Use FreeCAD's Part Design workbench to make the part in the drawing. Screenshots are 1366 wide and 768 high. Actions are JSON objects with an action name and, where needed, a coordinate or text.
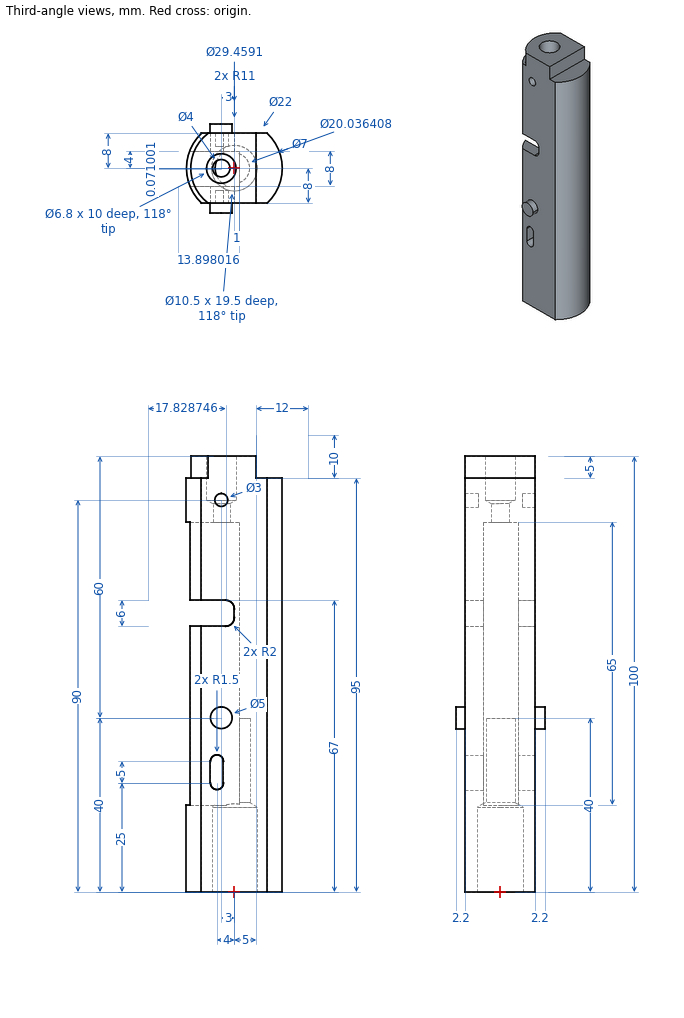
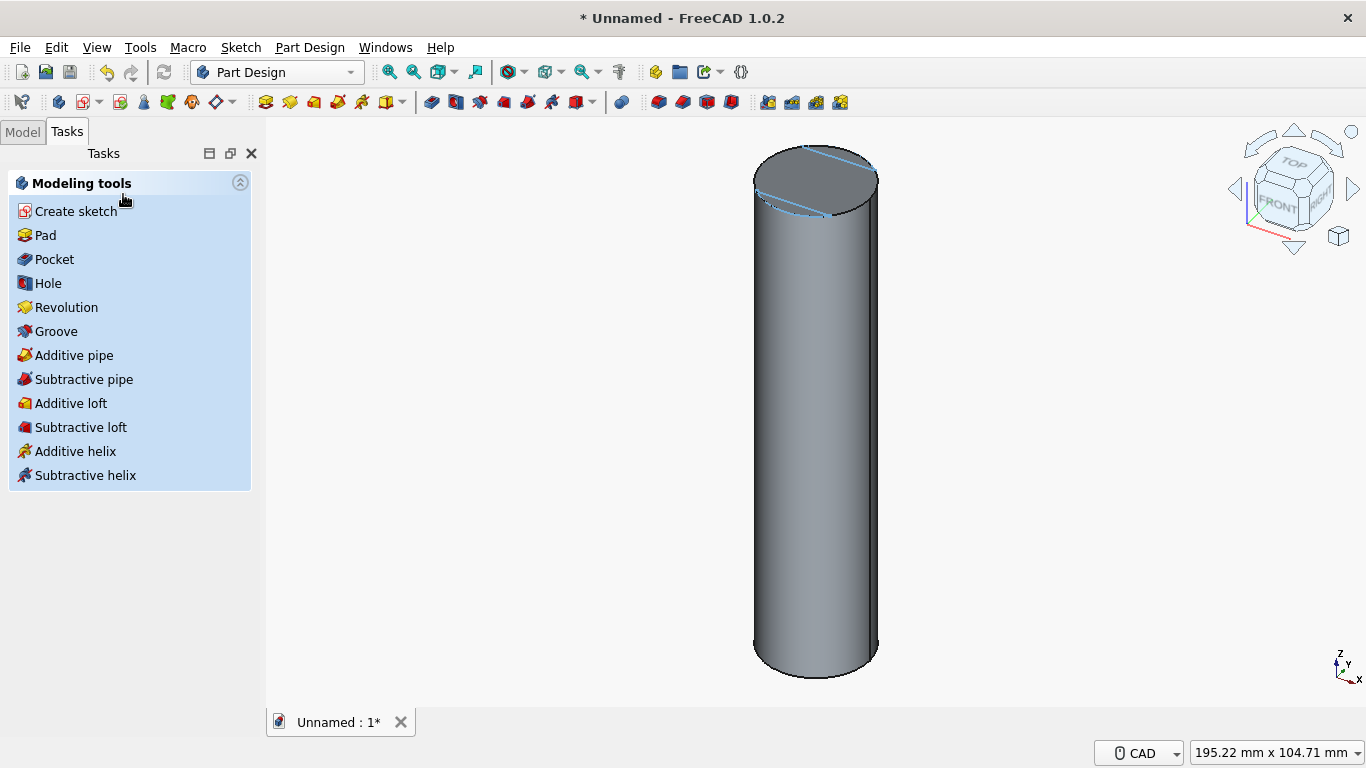
{"action": "left_click", "coordinate": [432, 102]}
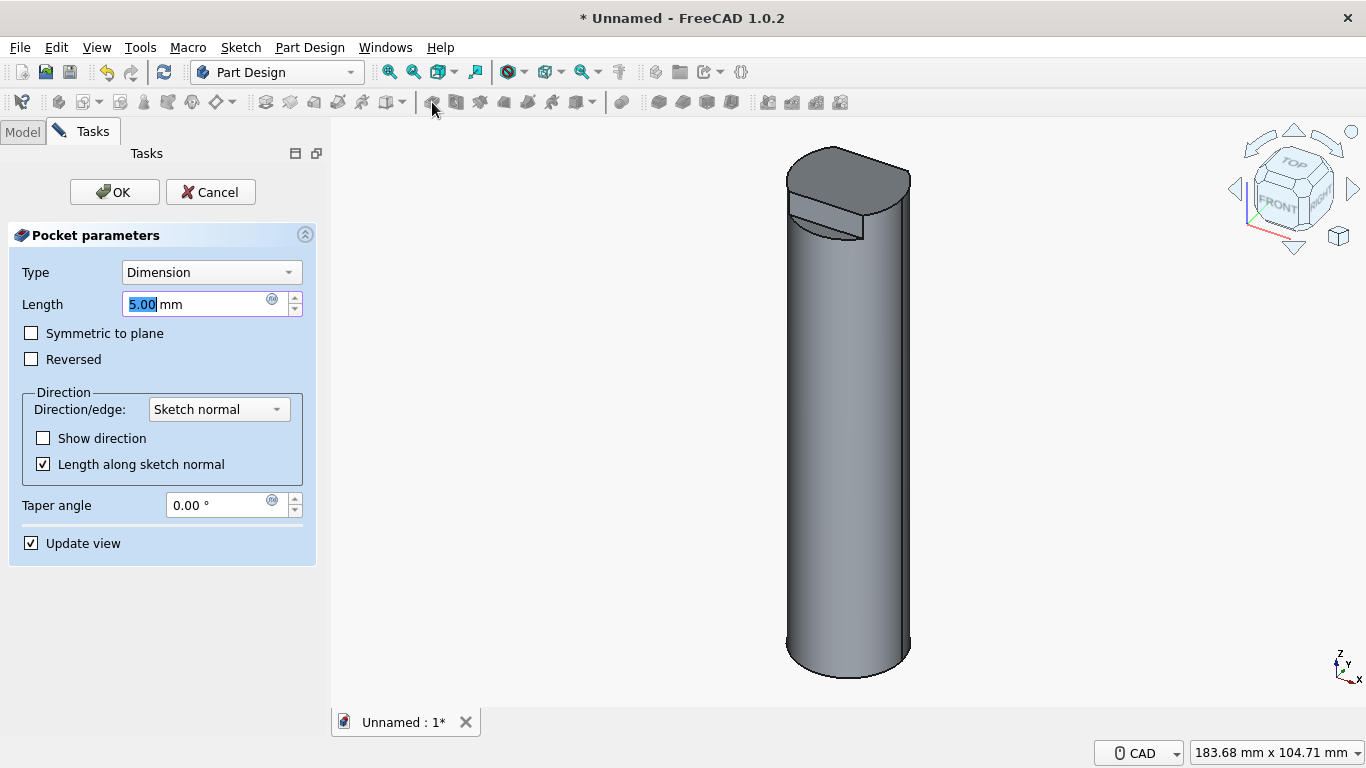
{"action": "left_click", "coordinate": [212, 272]}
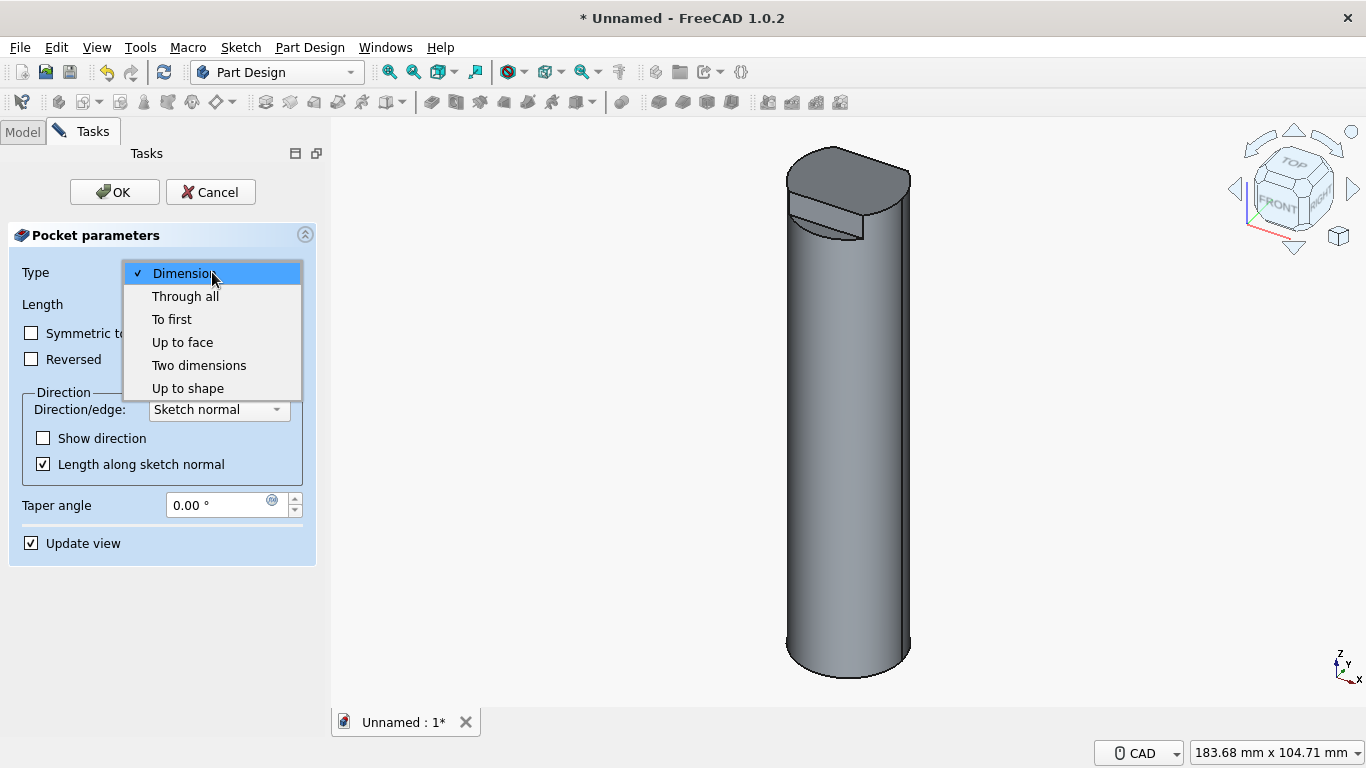
{"action": "left_click", "coordinate": [212, 296]}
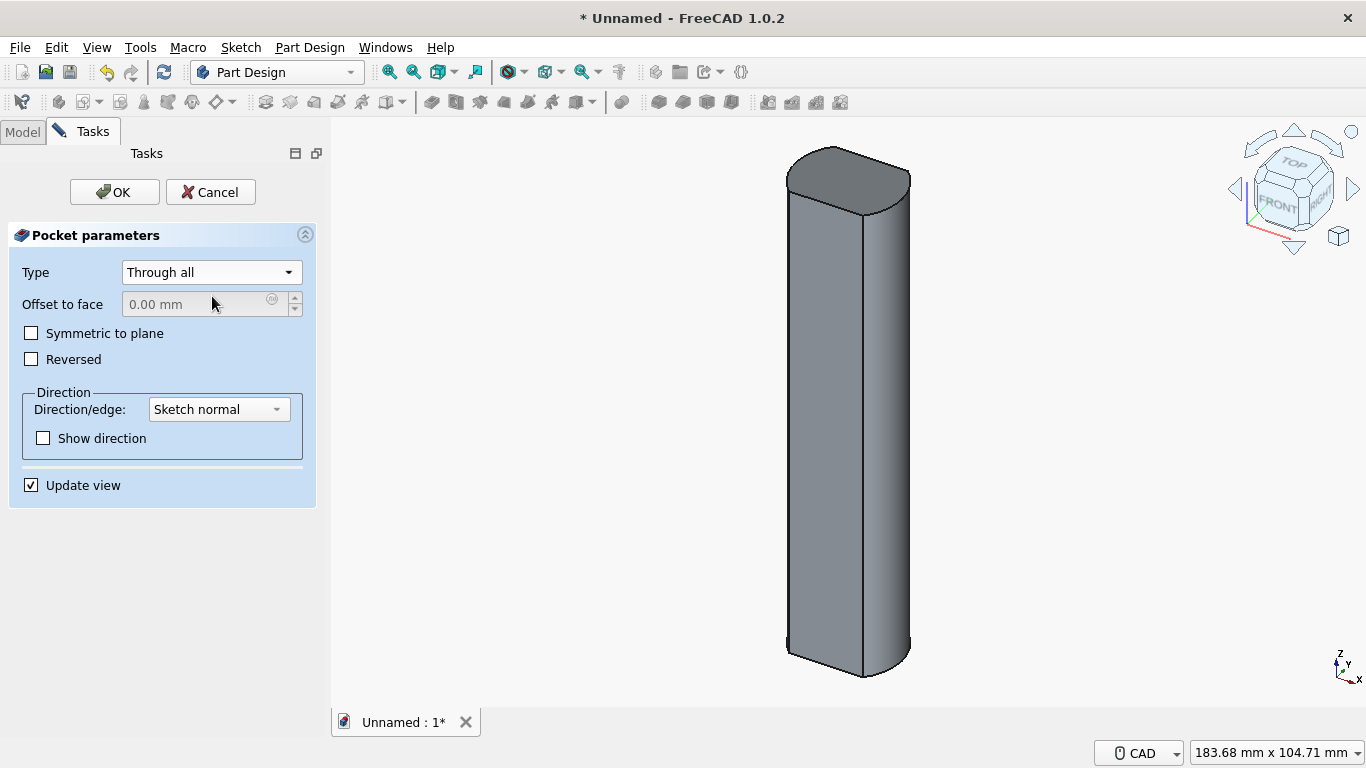
{"action": "left_click", "coordinate": [115, 192]}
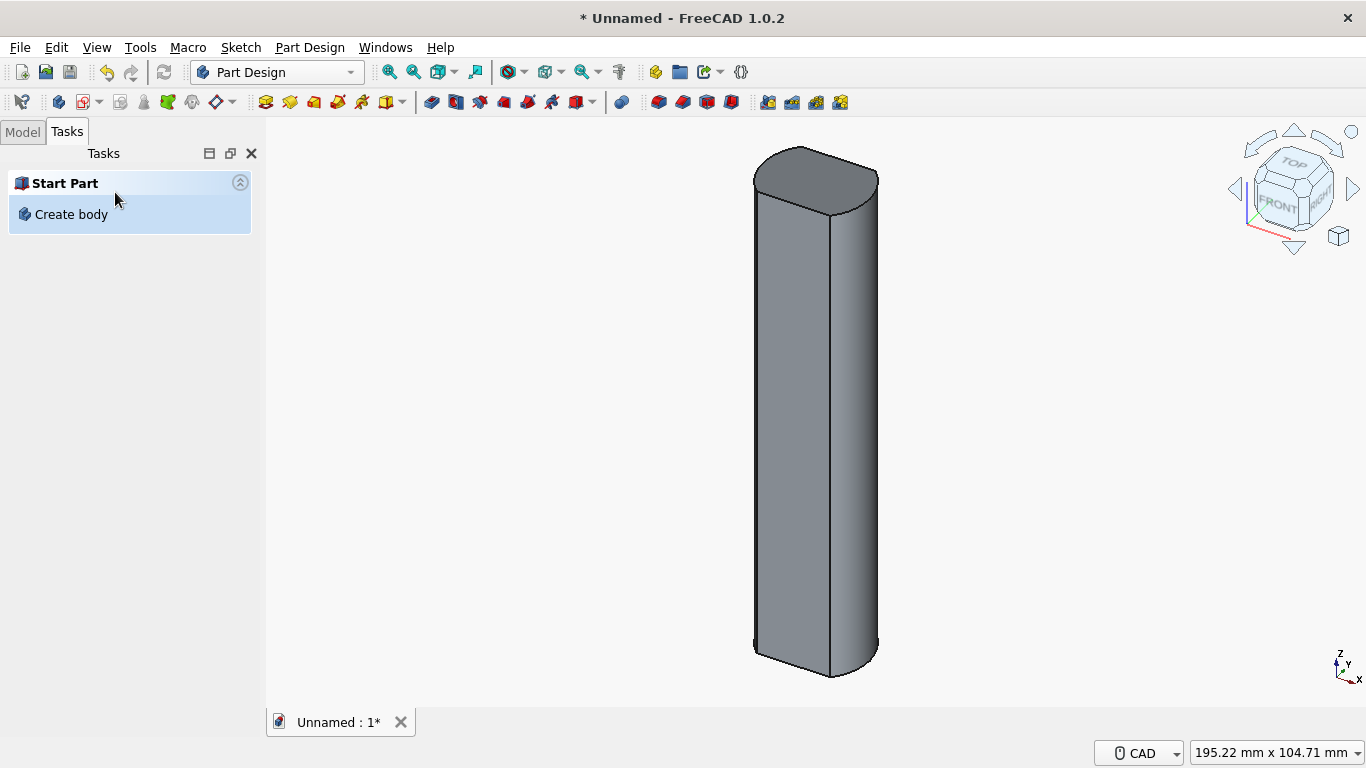
{"action": "left_click", "coordinate": [816, 180]}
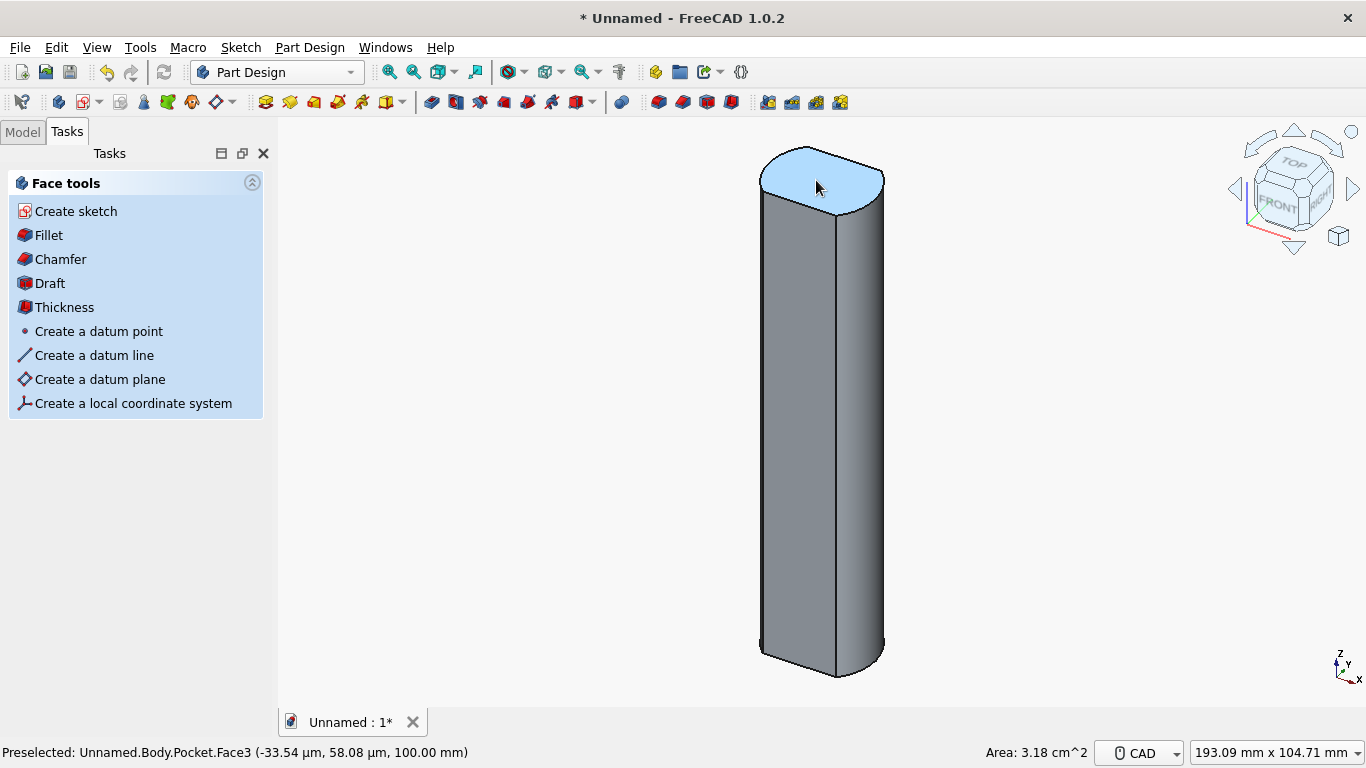
{"action": "left_click", "coordinate": [84, 102]}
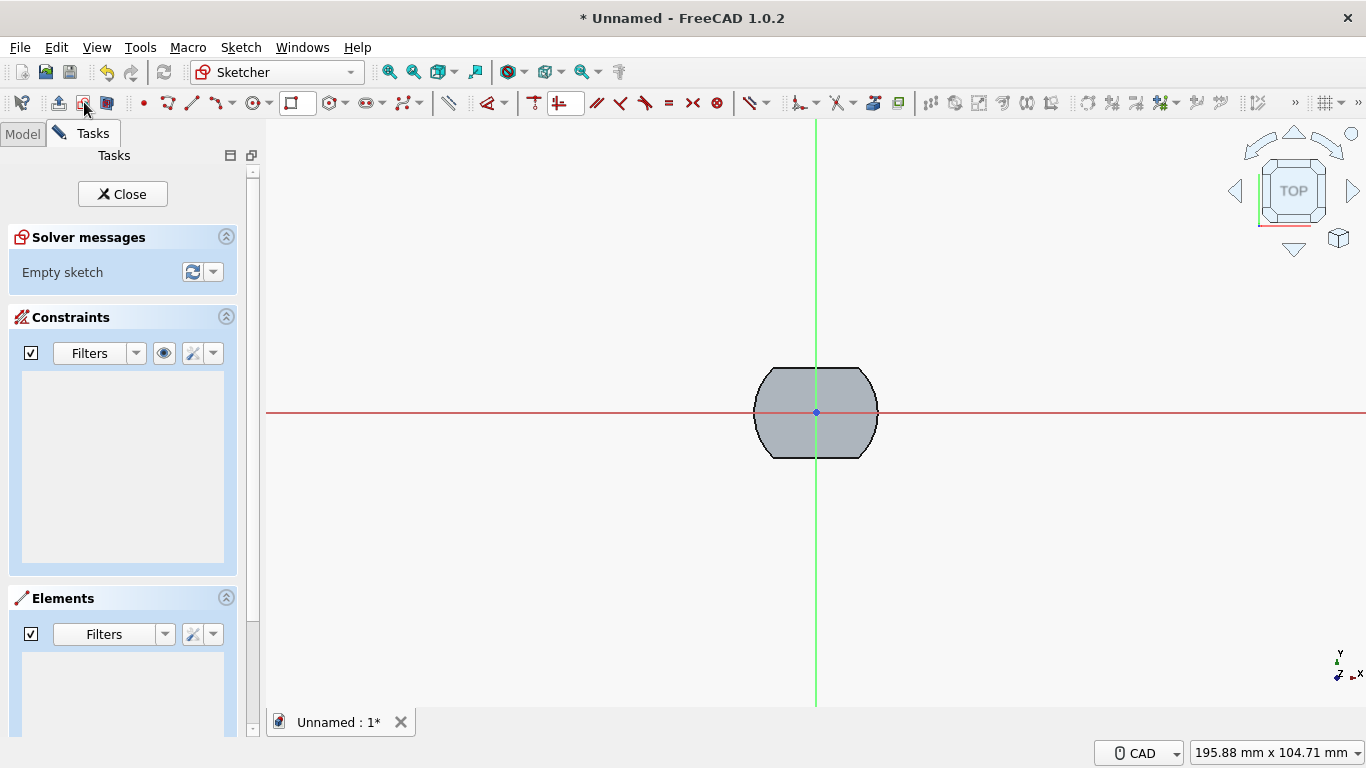
{"action": "scroll", "coordinate": [805, 413], "scroll_direction": "up", "scroll_amount": 14}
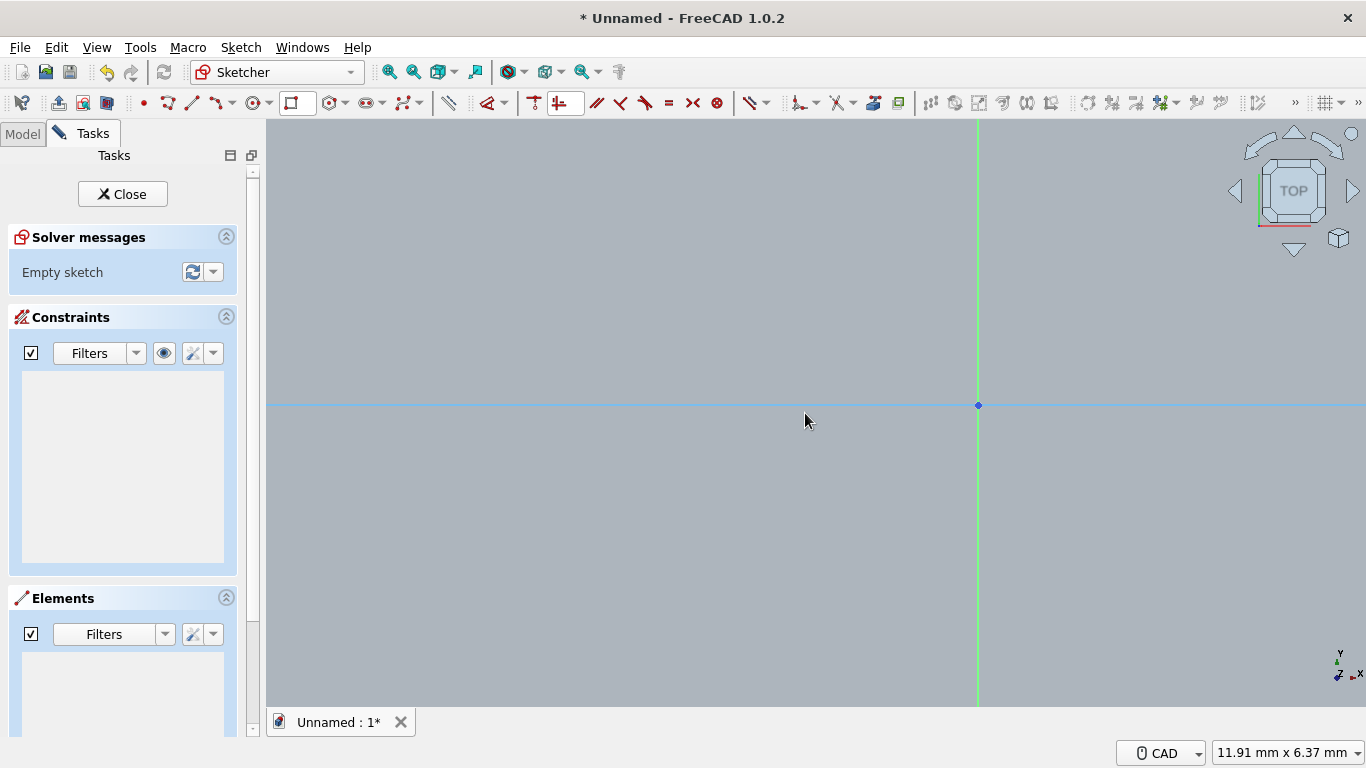
{"action": "key", "text": "g c"}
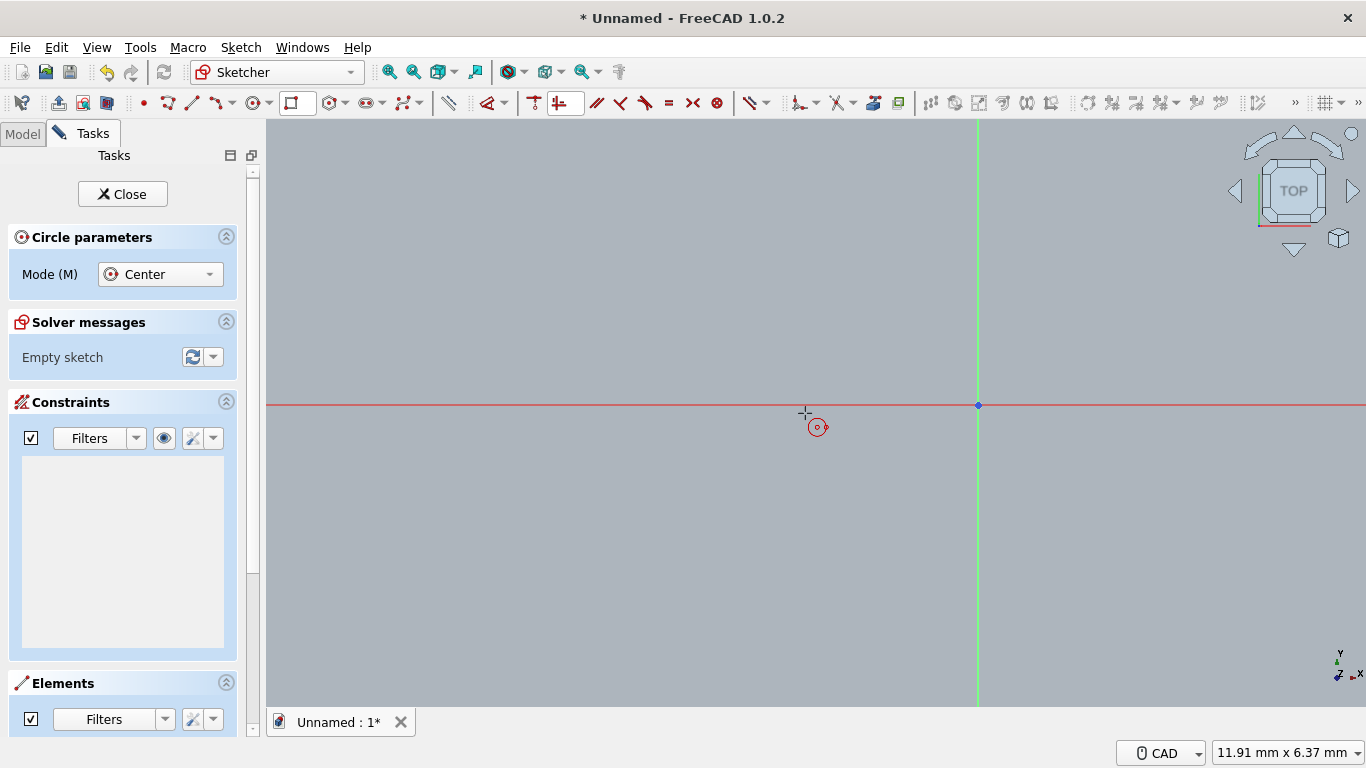
{"action": "left_click", "coordinate": [701, 405]}
{"action": "mouse_move", "coordinate": [832, 275]}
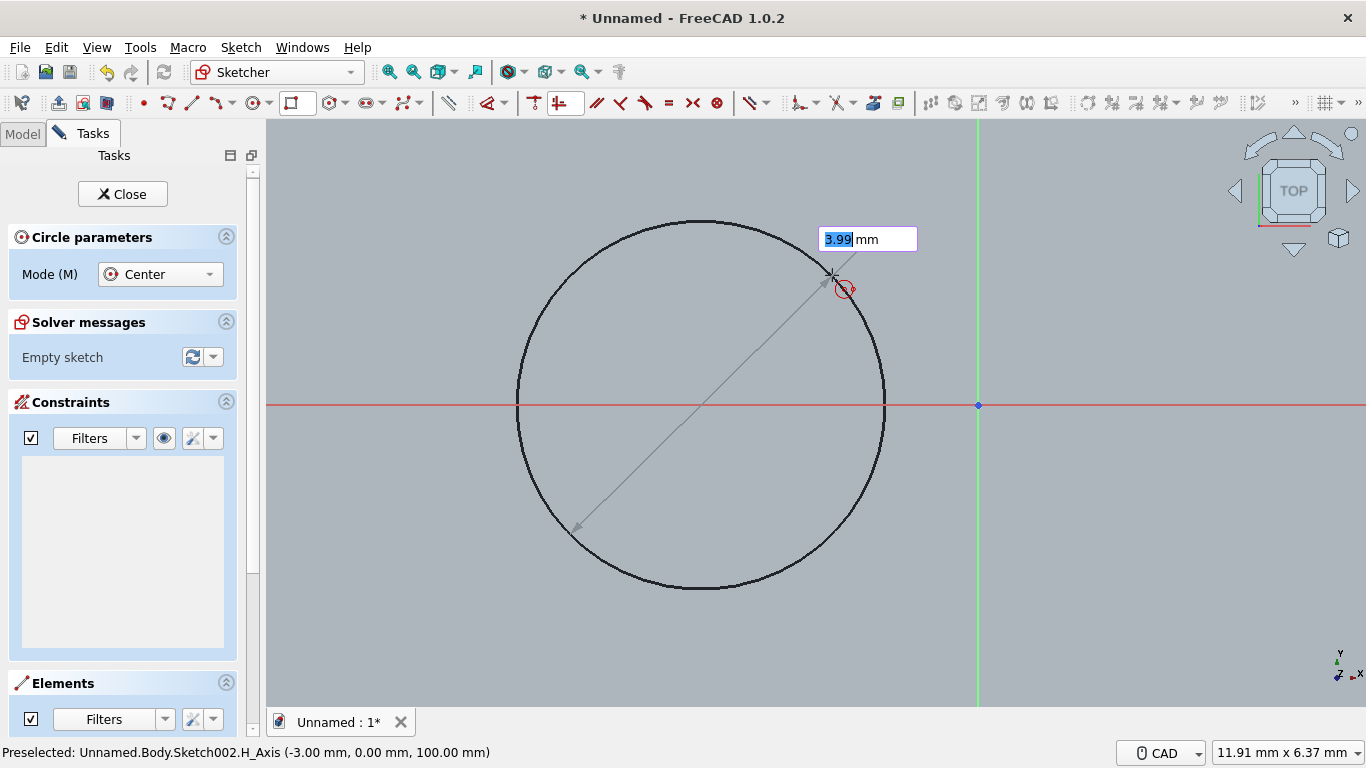
{"action": "type", "text": "4"}
{"action": "key", "text": "Return"}
{"action": "key", "text": "Escape"}